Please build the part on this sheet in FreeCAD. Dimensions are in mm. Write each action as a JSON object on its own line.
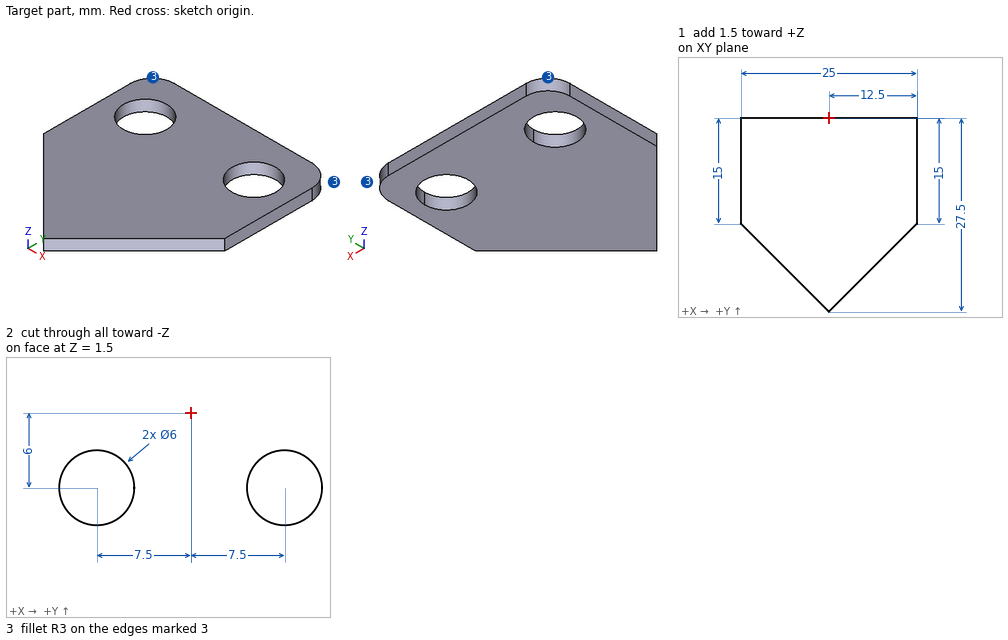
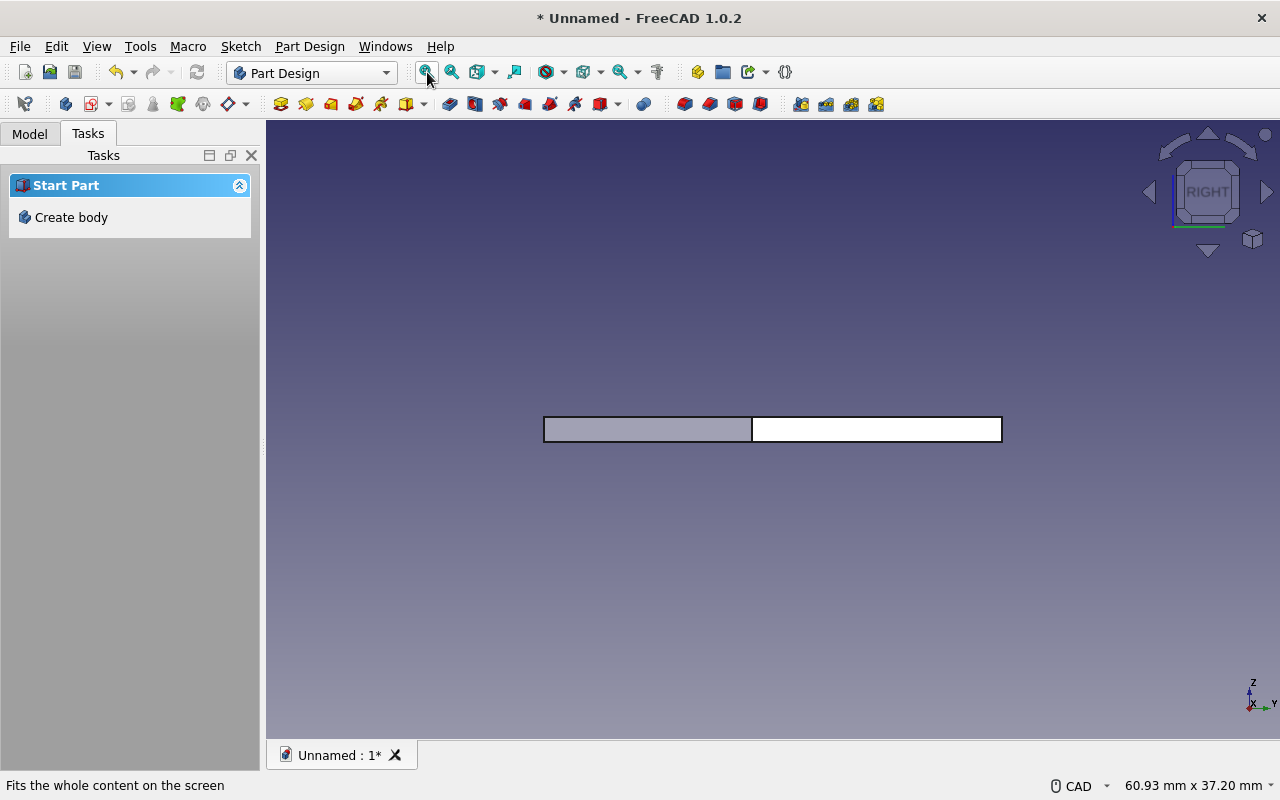
{"action": "left_click", "coordinate": [1002, 428]}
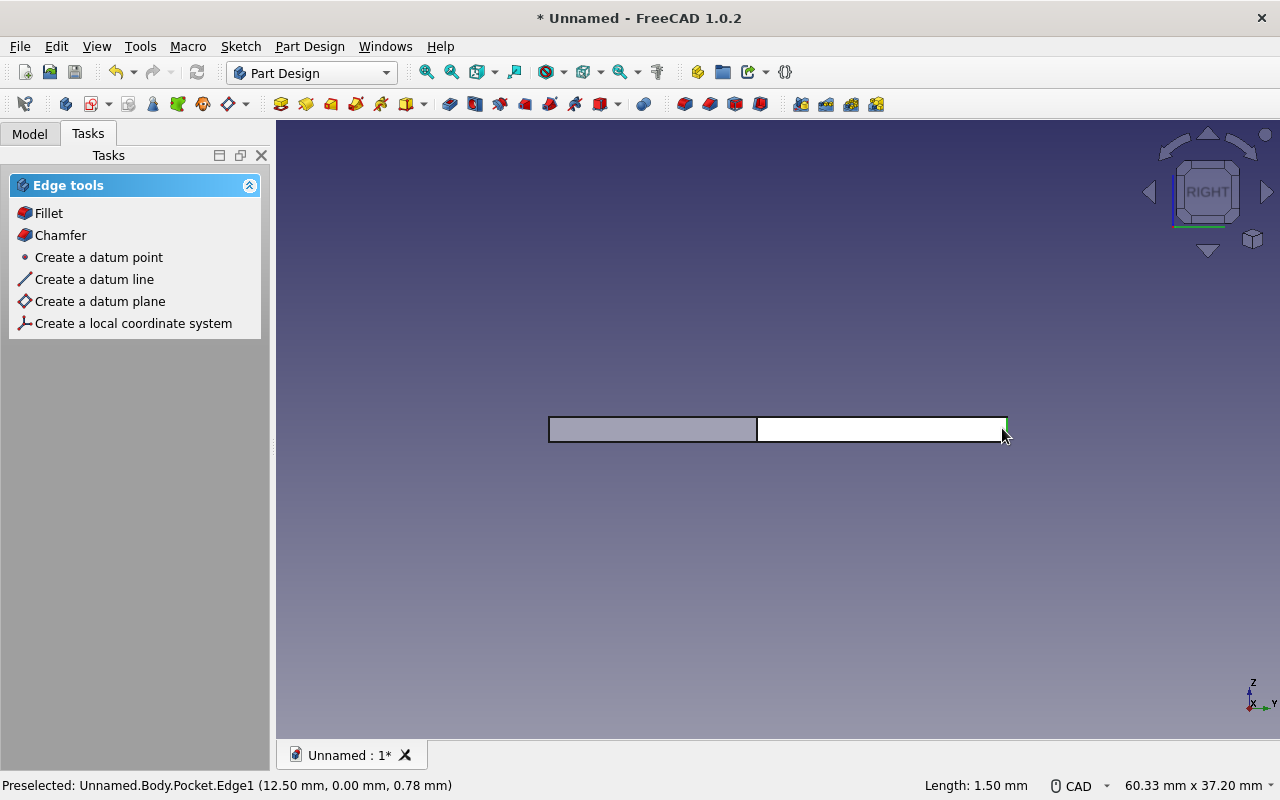
{"action": "key", "text": "5"}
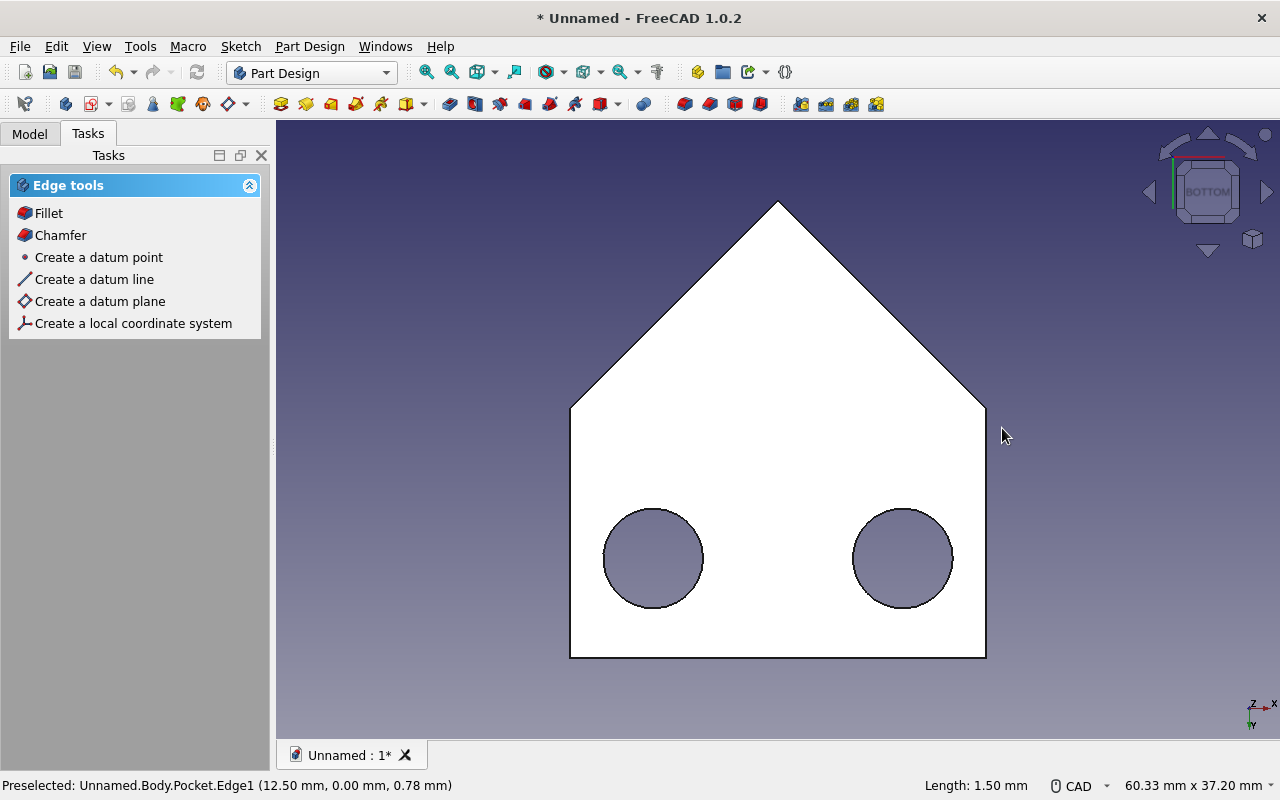
{"action": "key", "text": "4"}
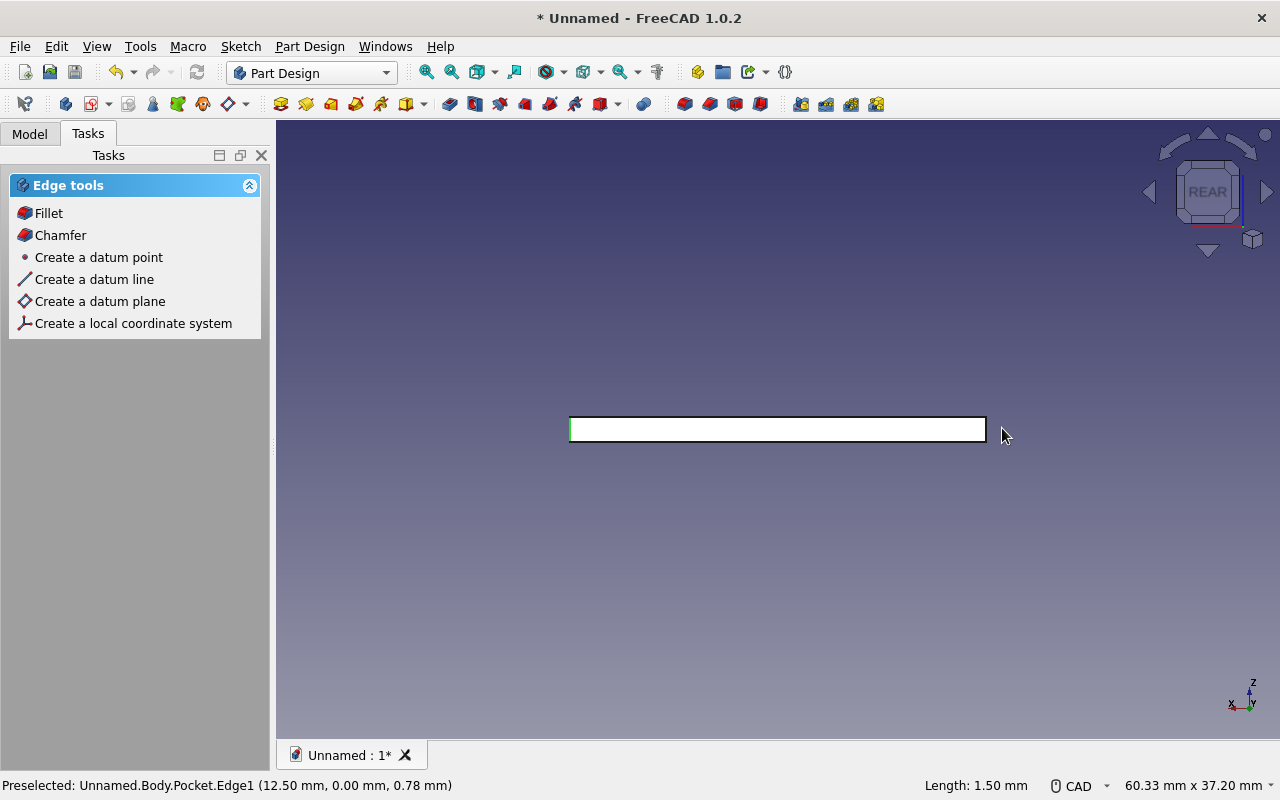
{"action": "left_click", "coordinate": [427, 72]}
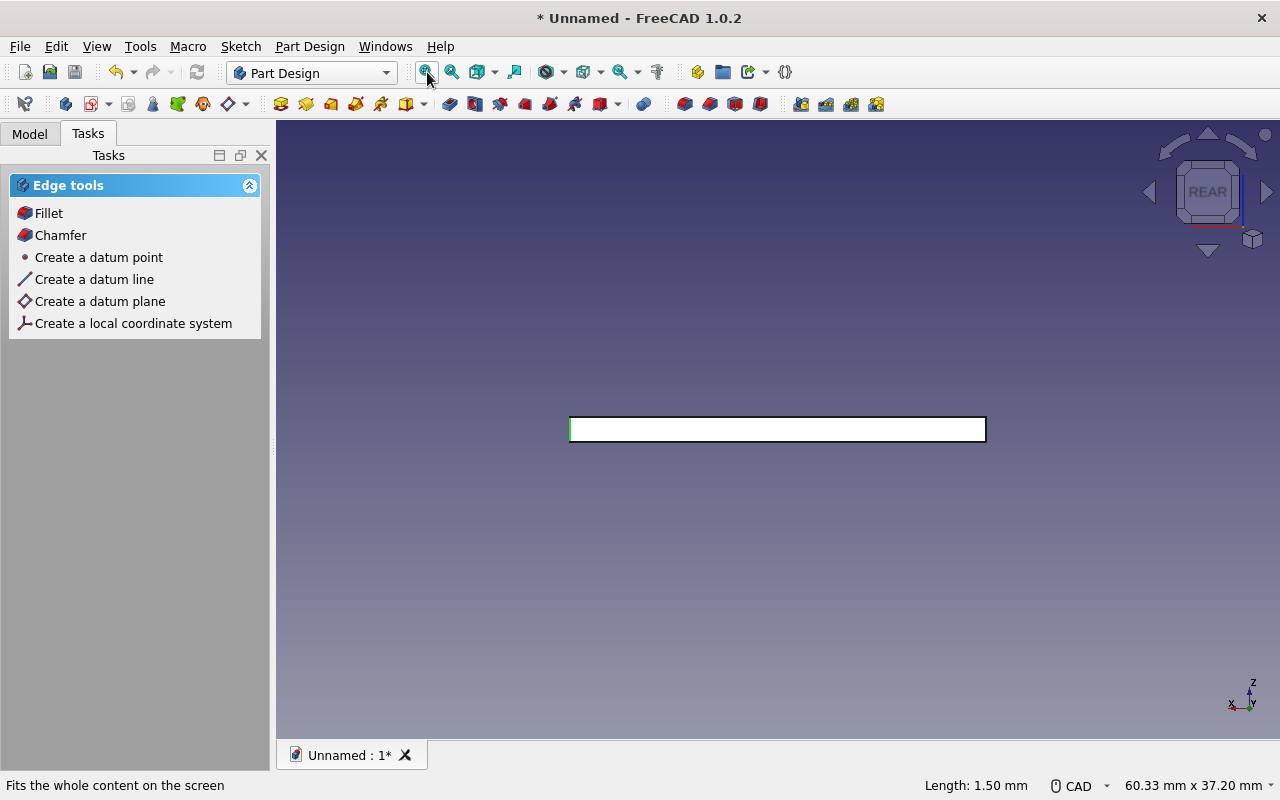
{"action": "left_click", "coordinate": [986, 429], "text": "ctrl"}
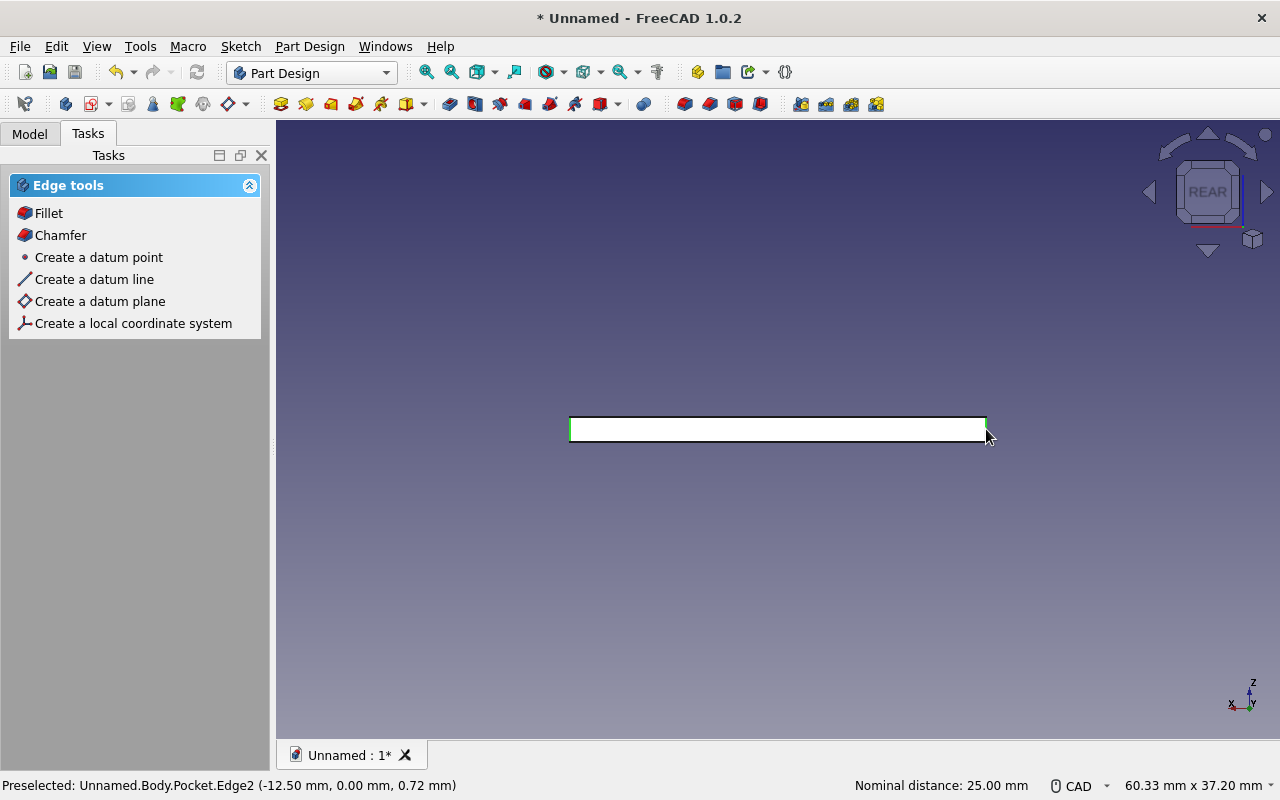
{"action": "left_click", "coordinate": [685, 104]}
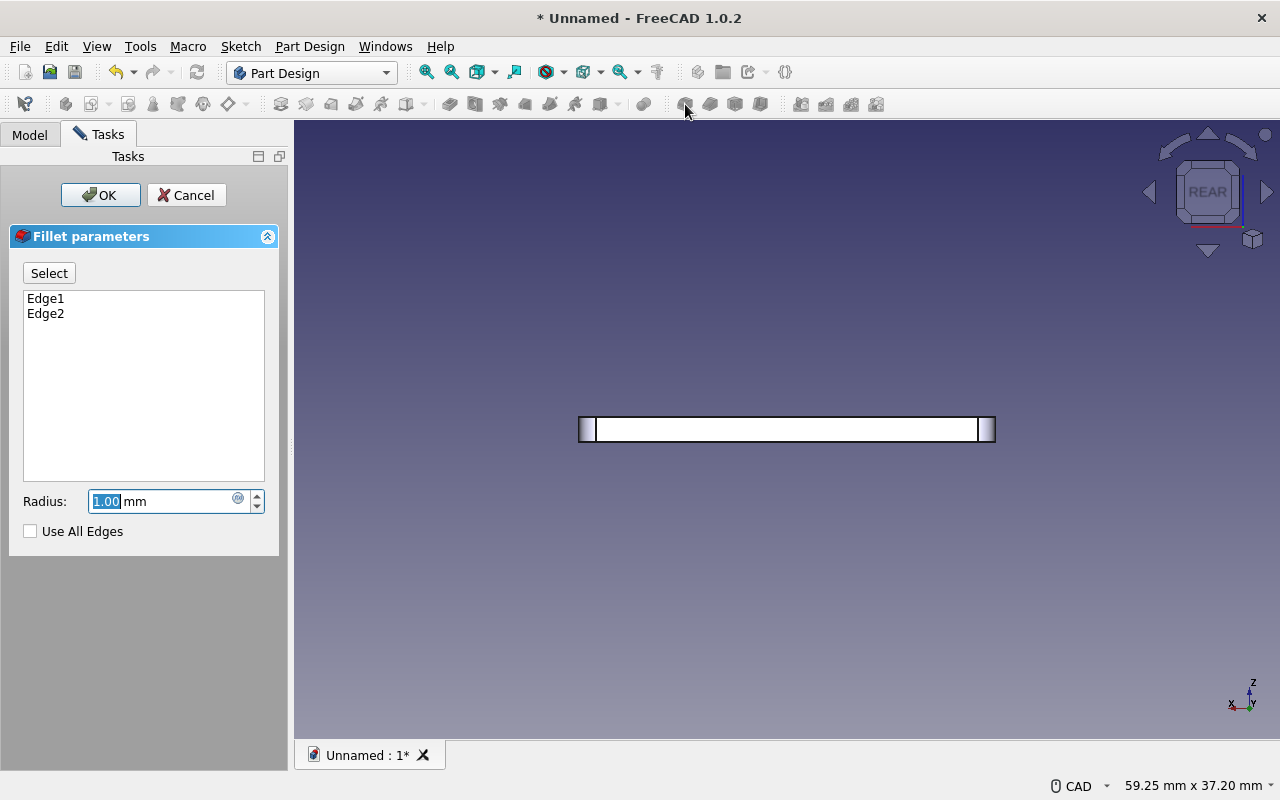
{"action": "type", "text": "3"}
{"action": "key", "text": "Tab"}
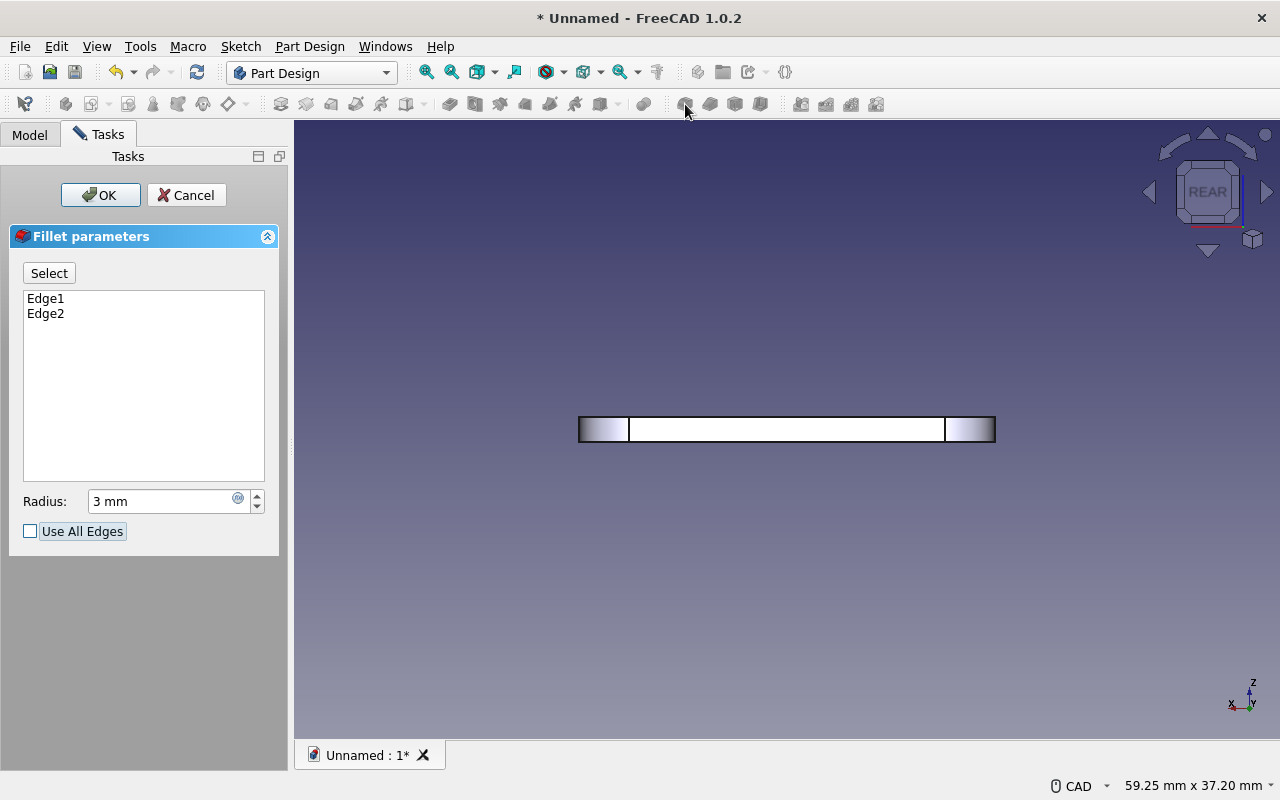
{"action": "left_click", "coordinate": [101, 195]}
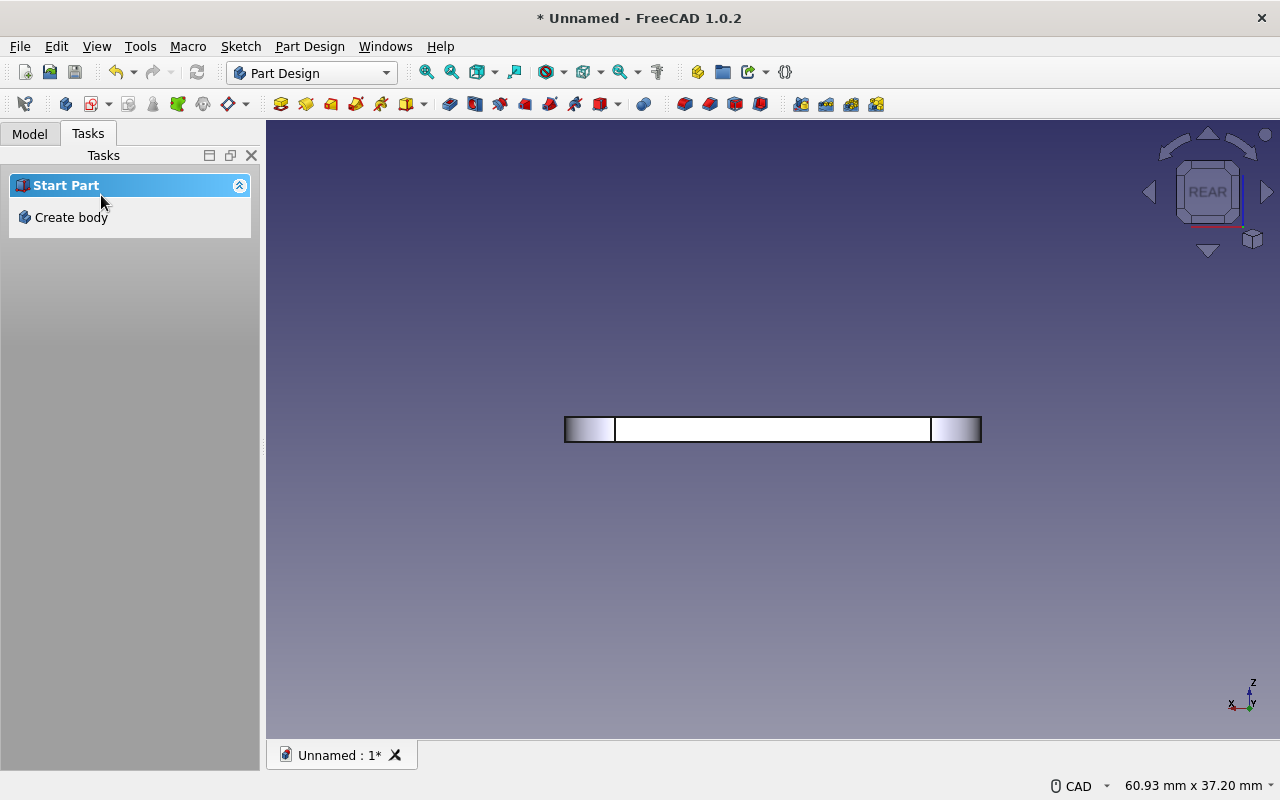
{"action": "key", "text": "0"}